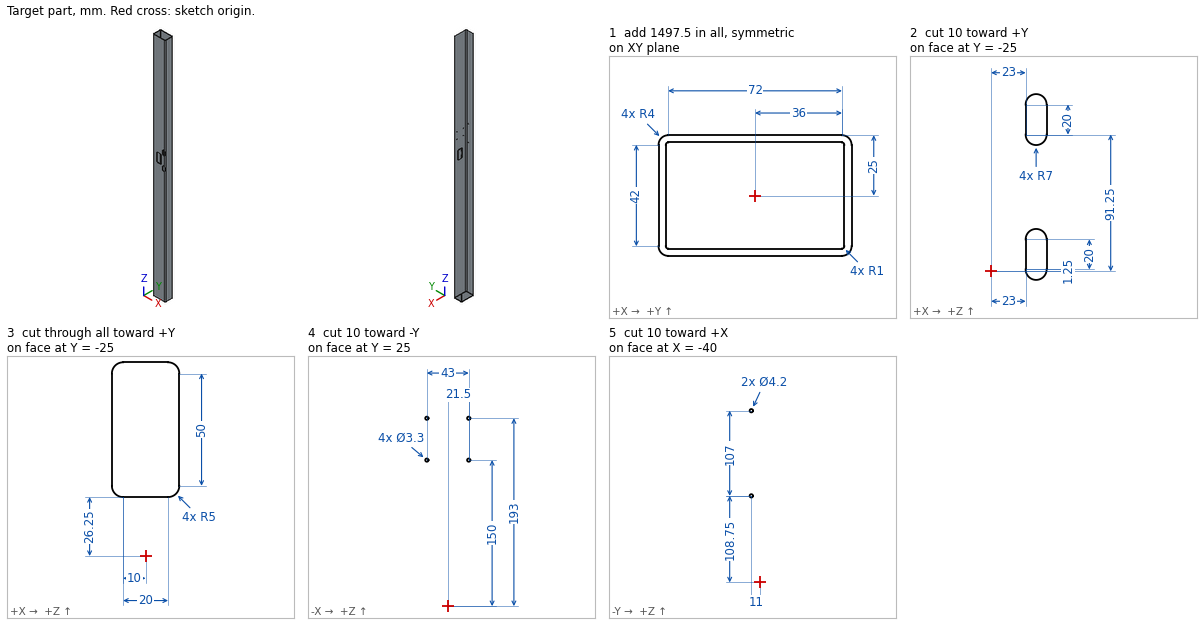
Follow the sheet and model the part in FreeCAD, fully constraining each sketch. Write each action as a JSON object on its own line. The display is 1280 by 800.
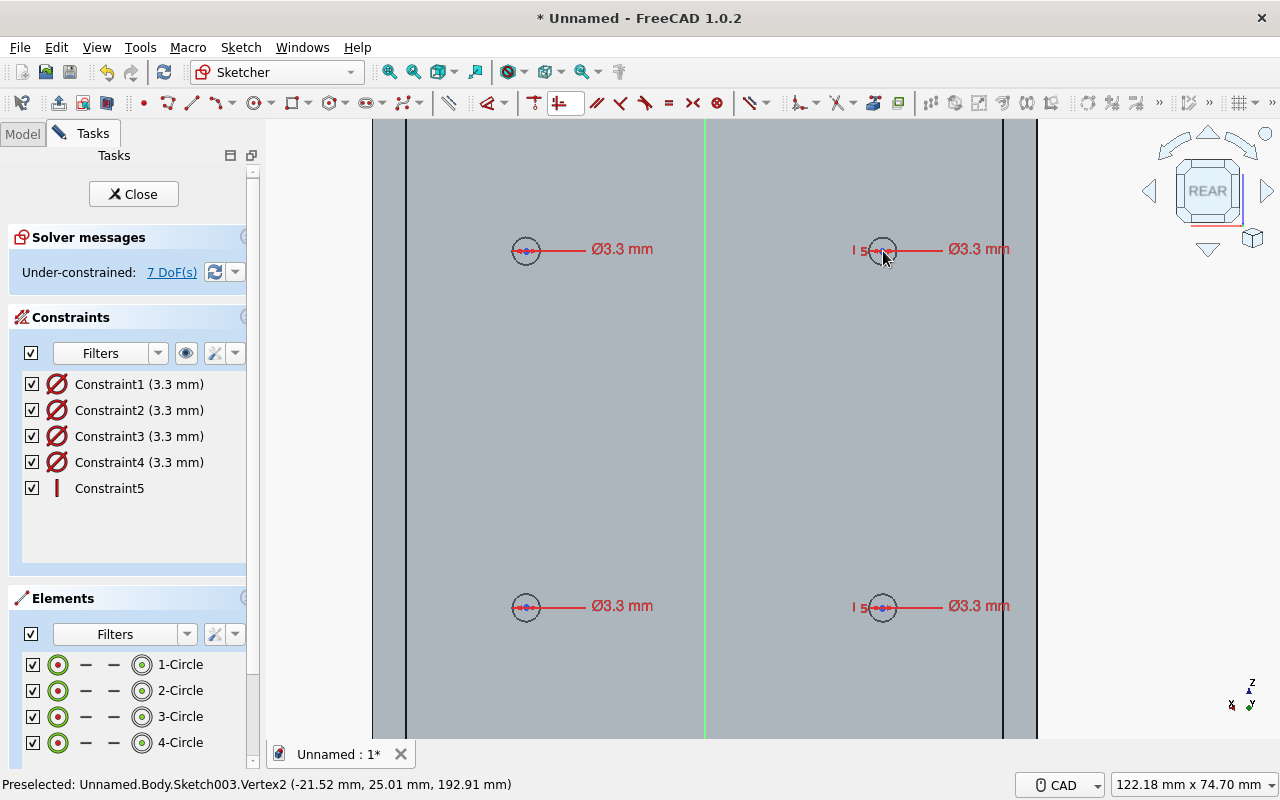
{"action": "left_click", "coordinate": [883, 608]}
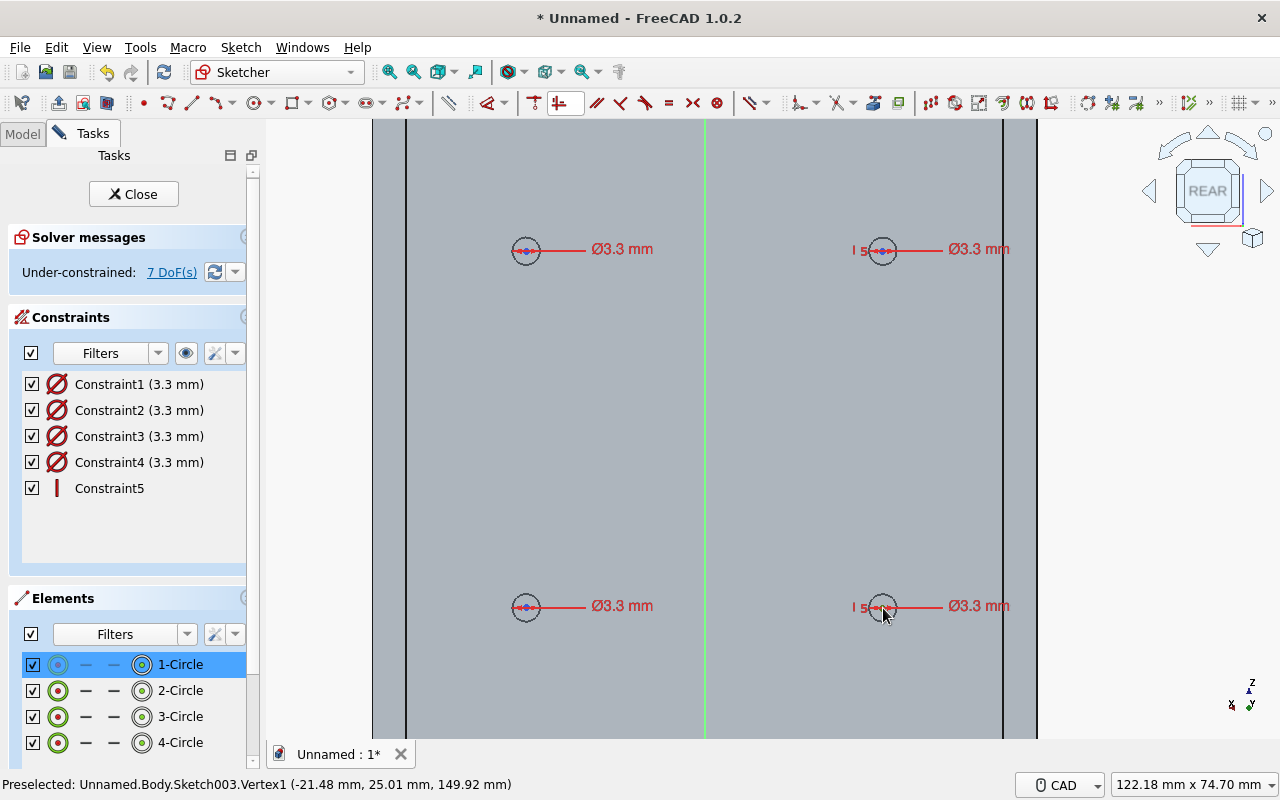
{"action": "left_click", "coordinate": [526, 608]}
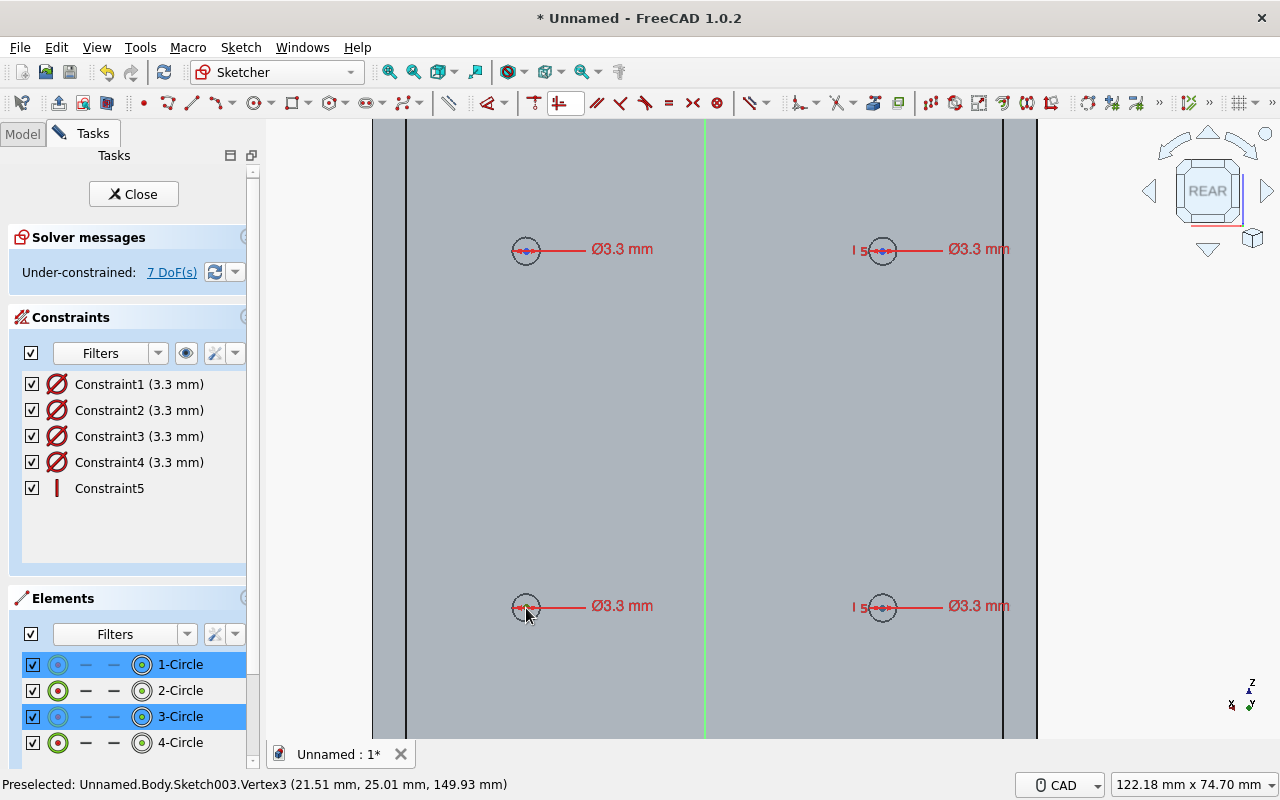
{"action": "left_click", "coordinate": [578, 104]}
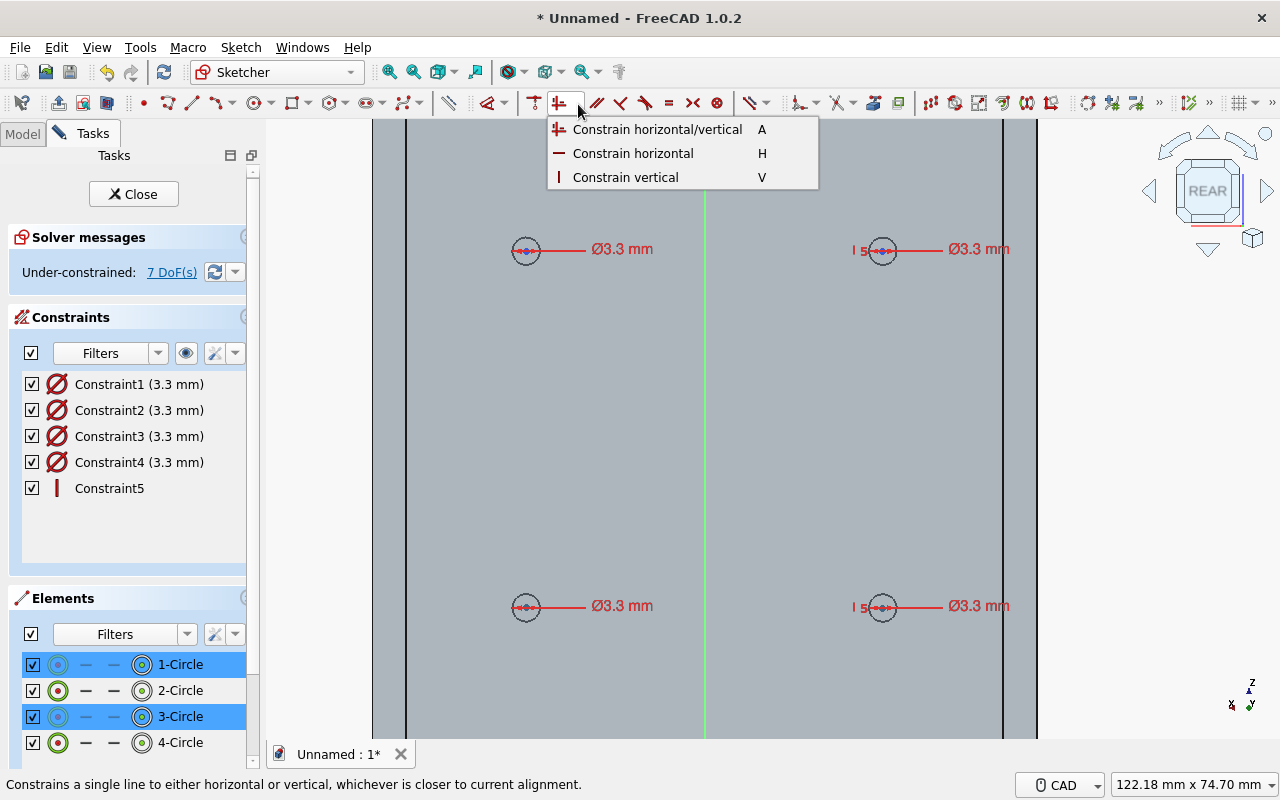
{"action": "left_click", "coordinate": [683, 153]}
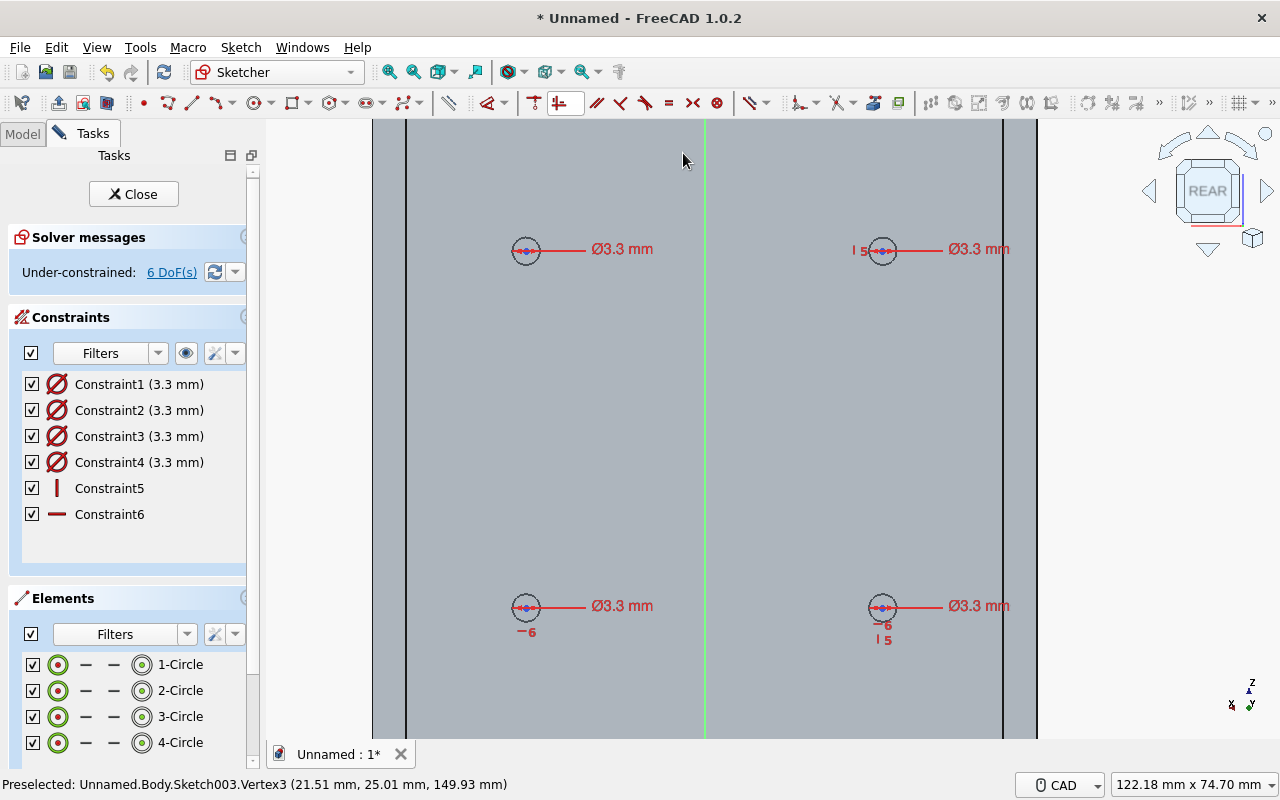
{"action": "left_click", "coordinate": [526, 608]}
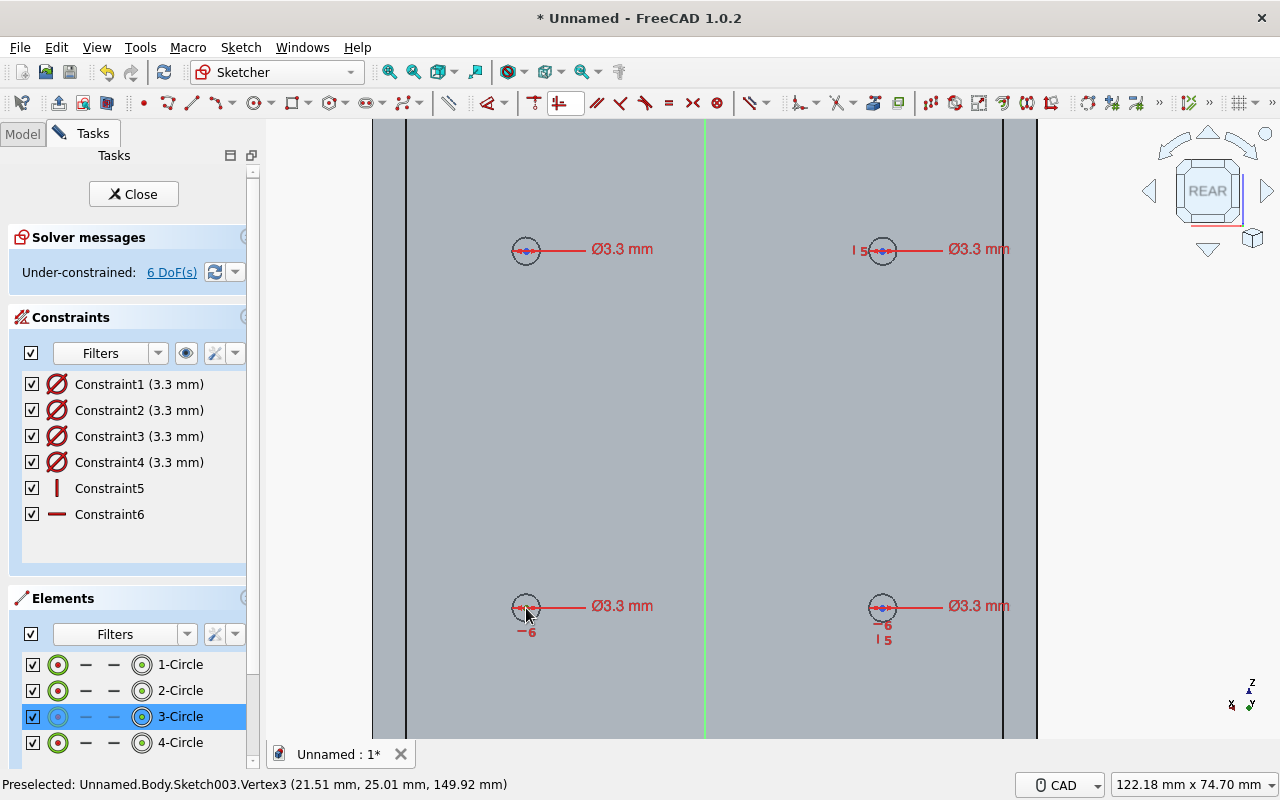
{"action": "left_click", "coordinate": [526, 251]}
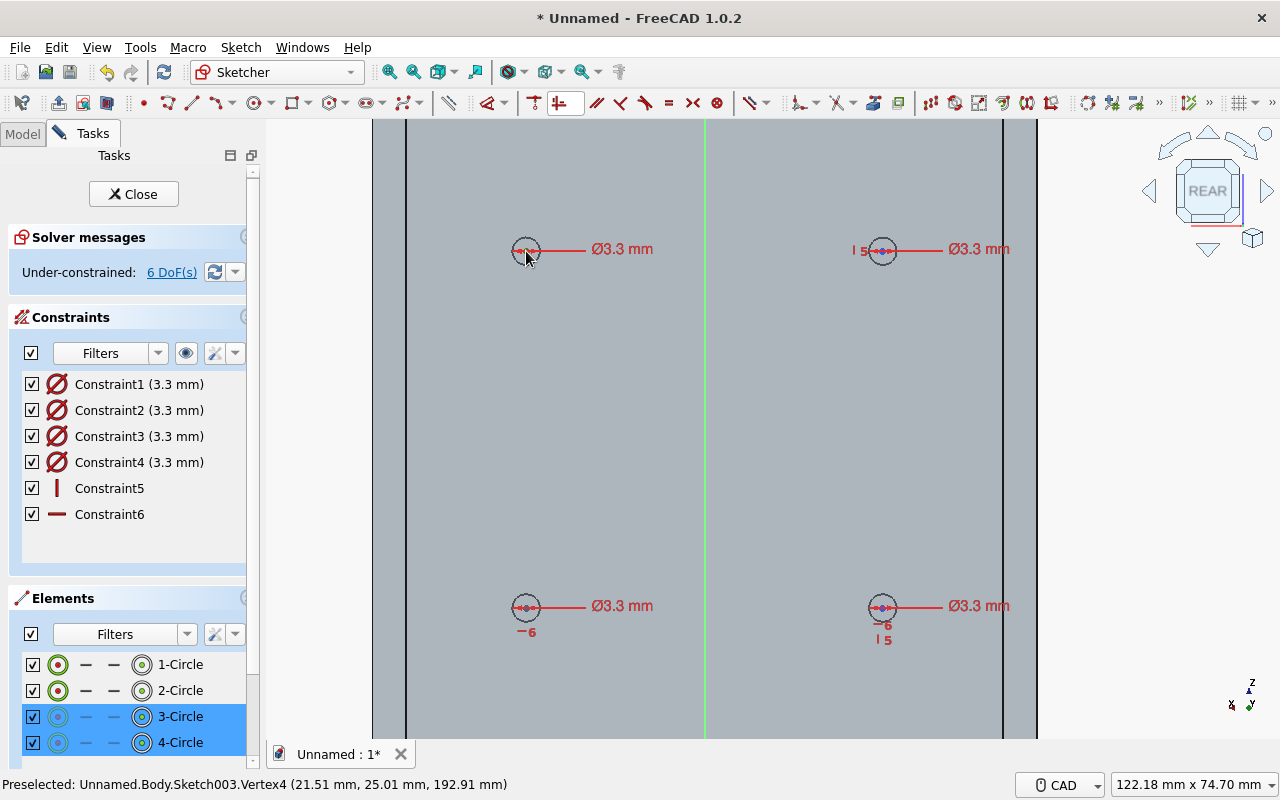
{"action": "key", "text": "v"}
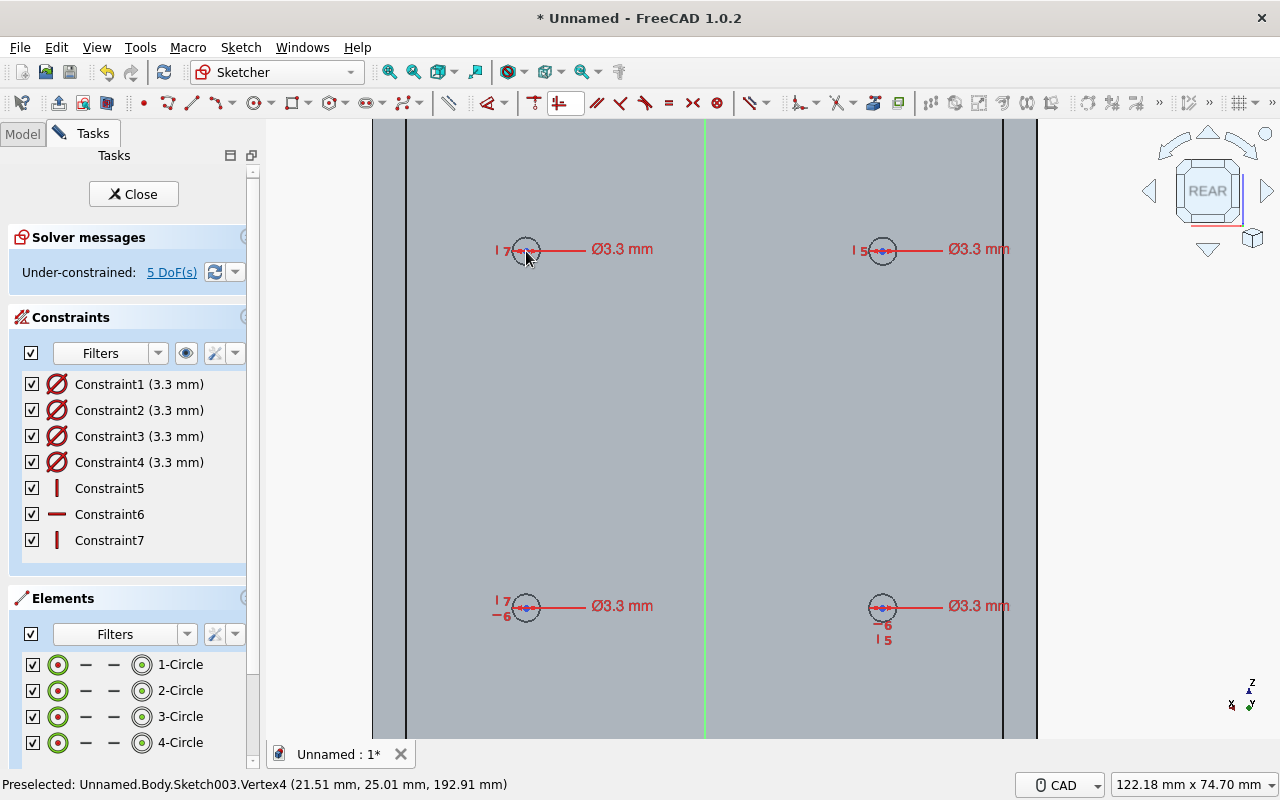
{"action": "left_click", "coordinate": [883, 251]}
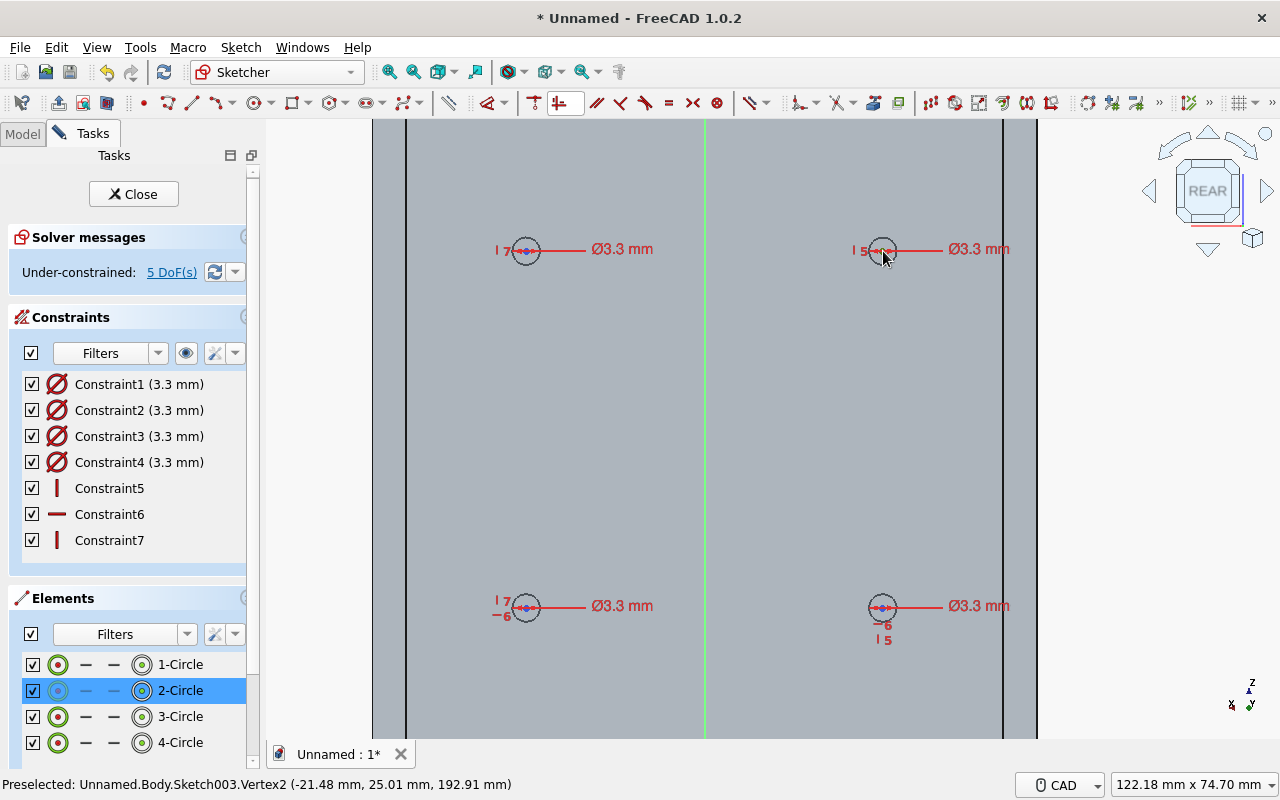
{"action": "left_click", "coordinate": [526, 251]}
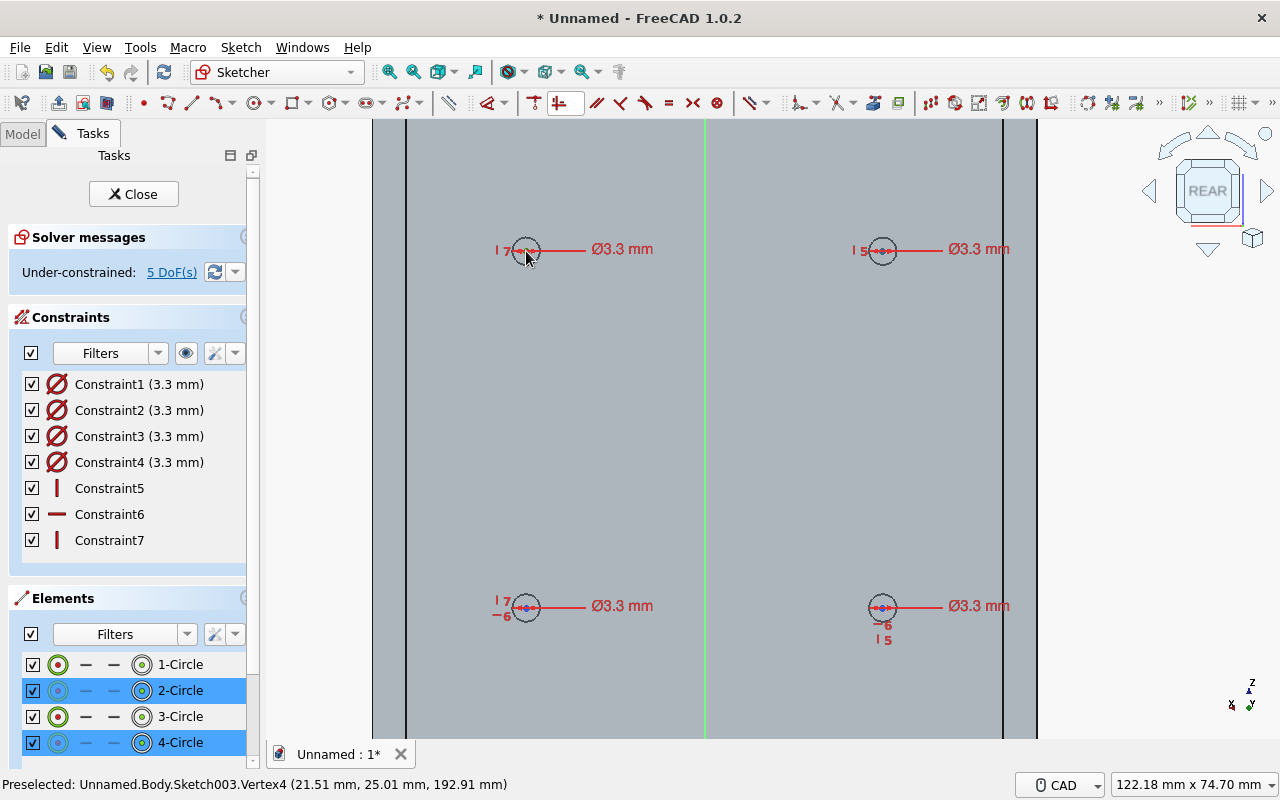
{"action": "left_click", "coordinate": [578, 104]}